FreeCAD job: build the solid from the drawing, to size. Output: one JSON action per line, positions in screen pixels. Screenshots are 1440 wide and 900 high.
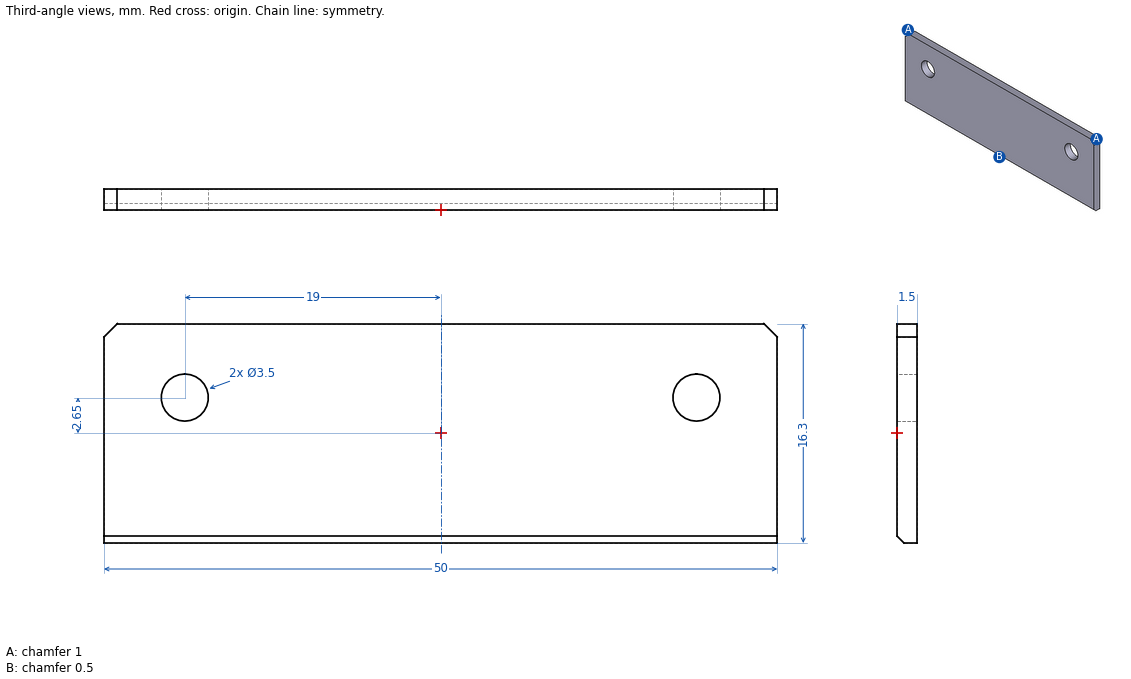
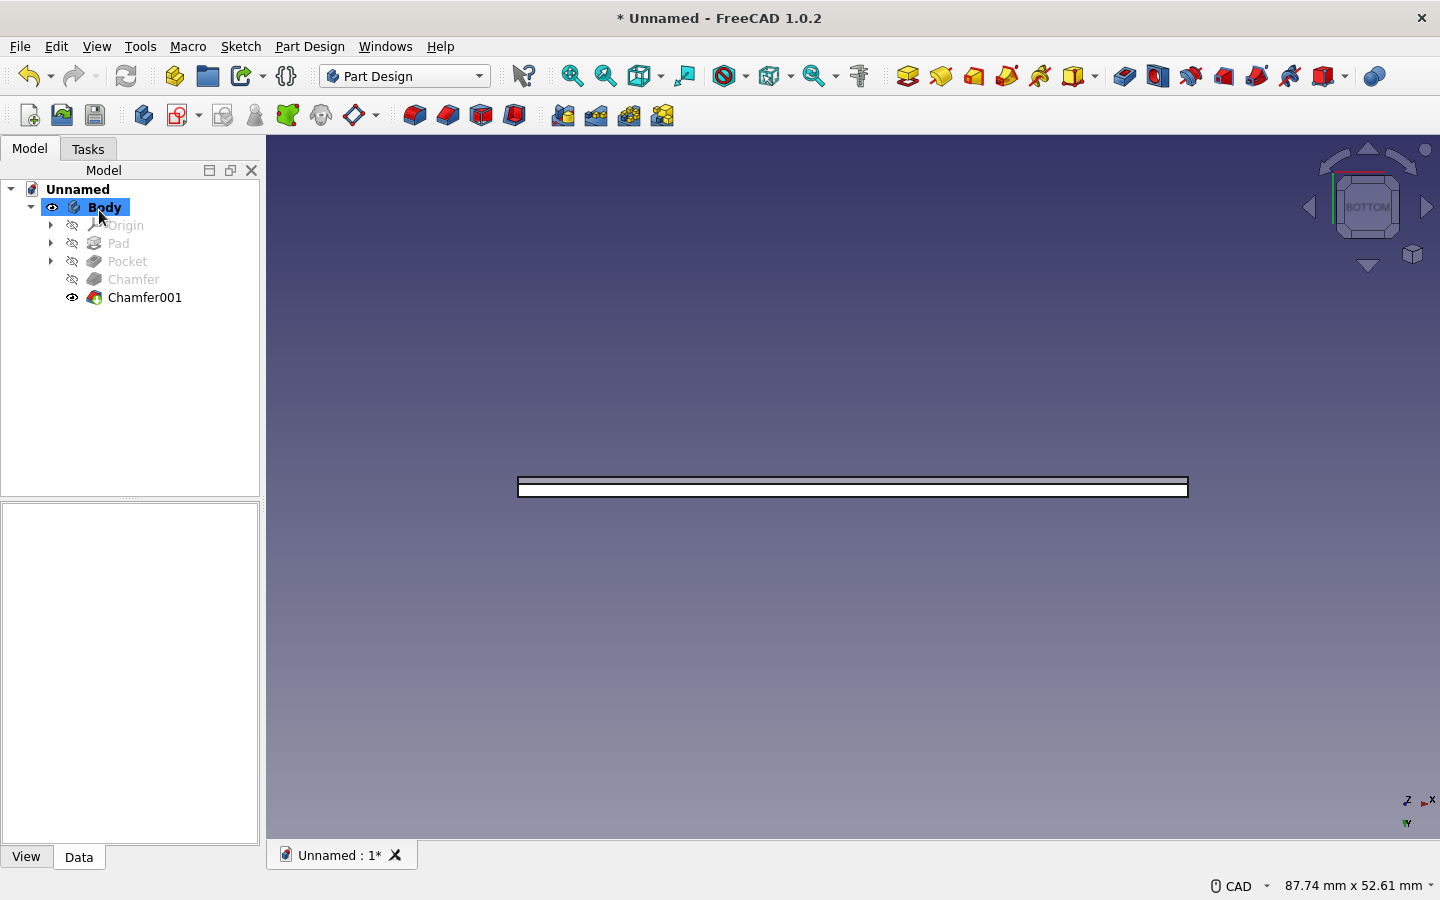
{"action": "key", "text": "0"}